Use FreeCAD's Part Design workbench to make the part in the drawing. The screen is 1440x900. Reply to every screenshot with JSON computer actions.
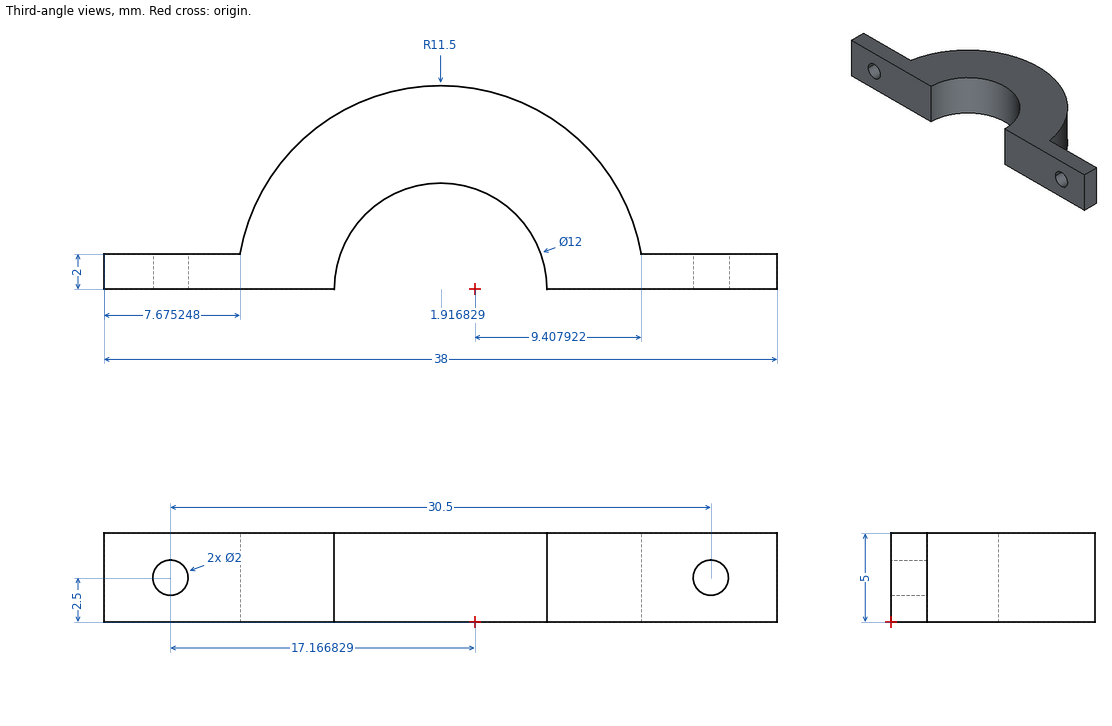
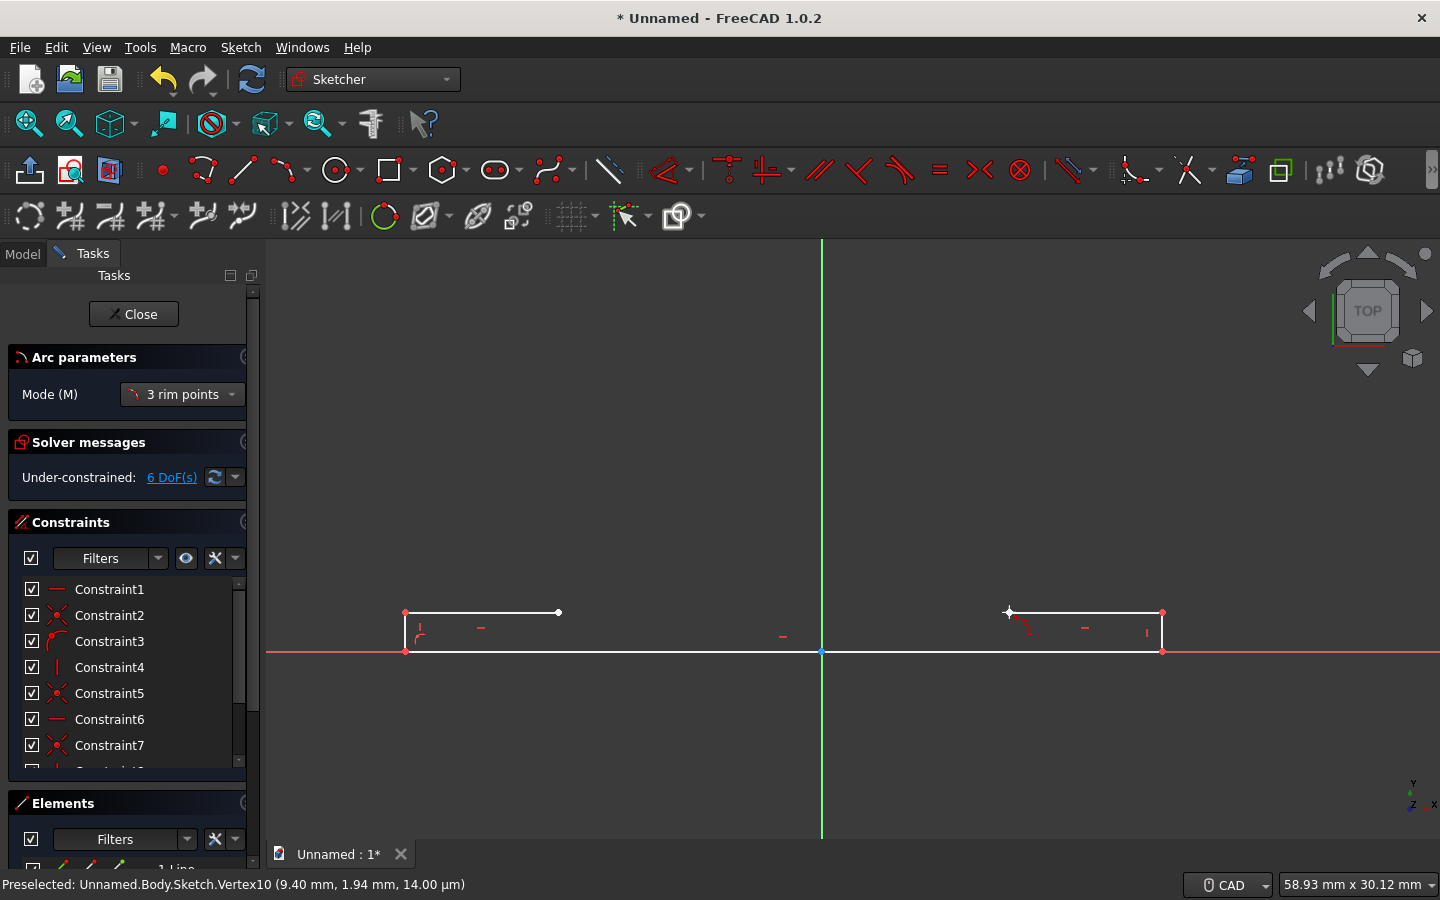
{"action": "left_click", "coordinate": [1009, 613]}
{"action": "left_click", "coordinate": [558, 613]}
{"action": "left_click", "coordinate": [783, 423]}
{"action": "key", "text": "Escape"}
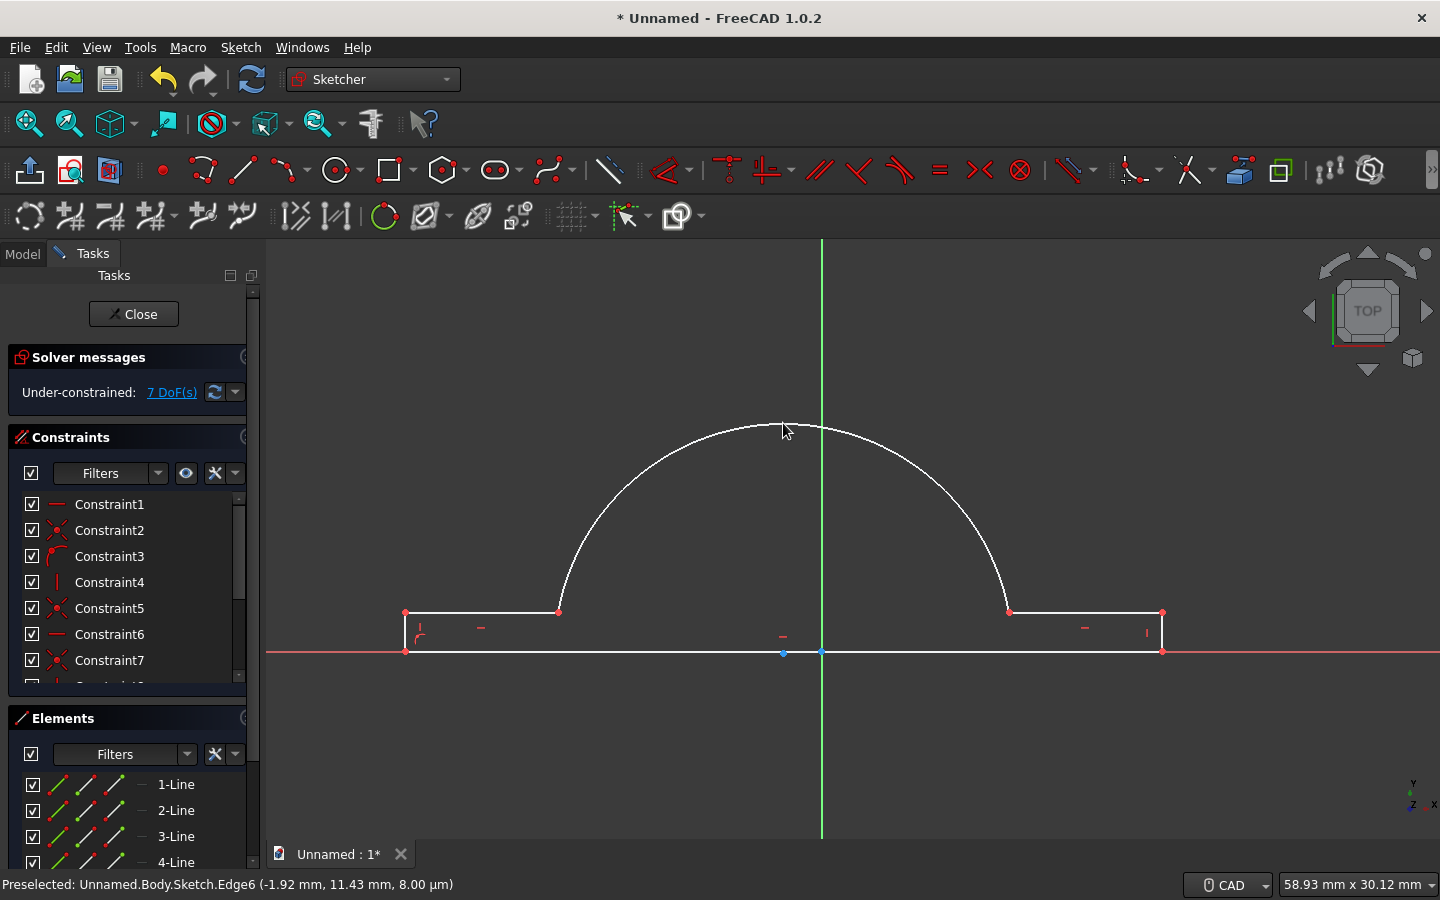
{"action": "left_click", "coordinate": [784, 653]}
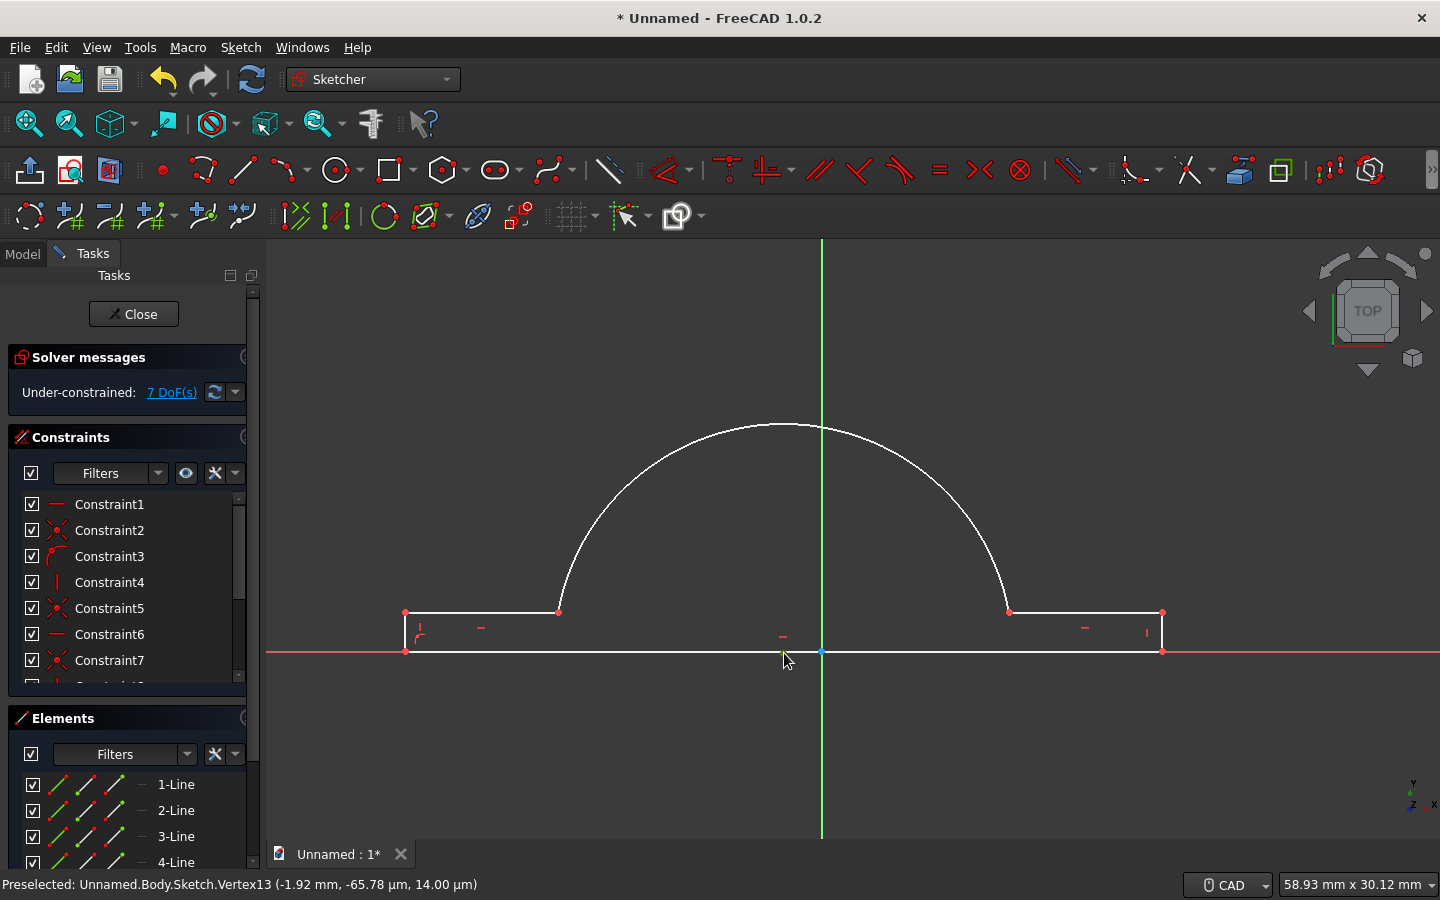
{"action": "left_click", "coordinate": [364, 652]}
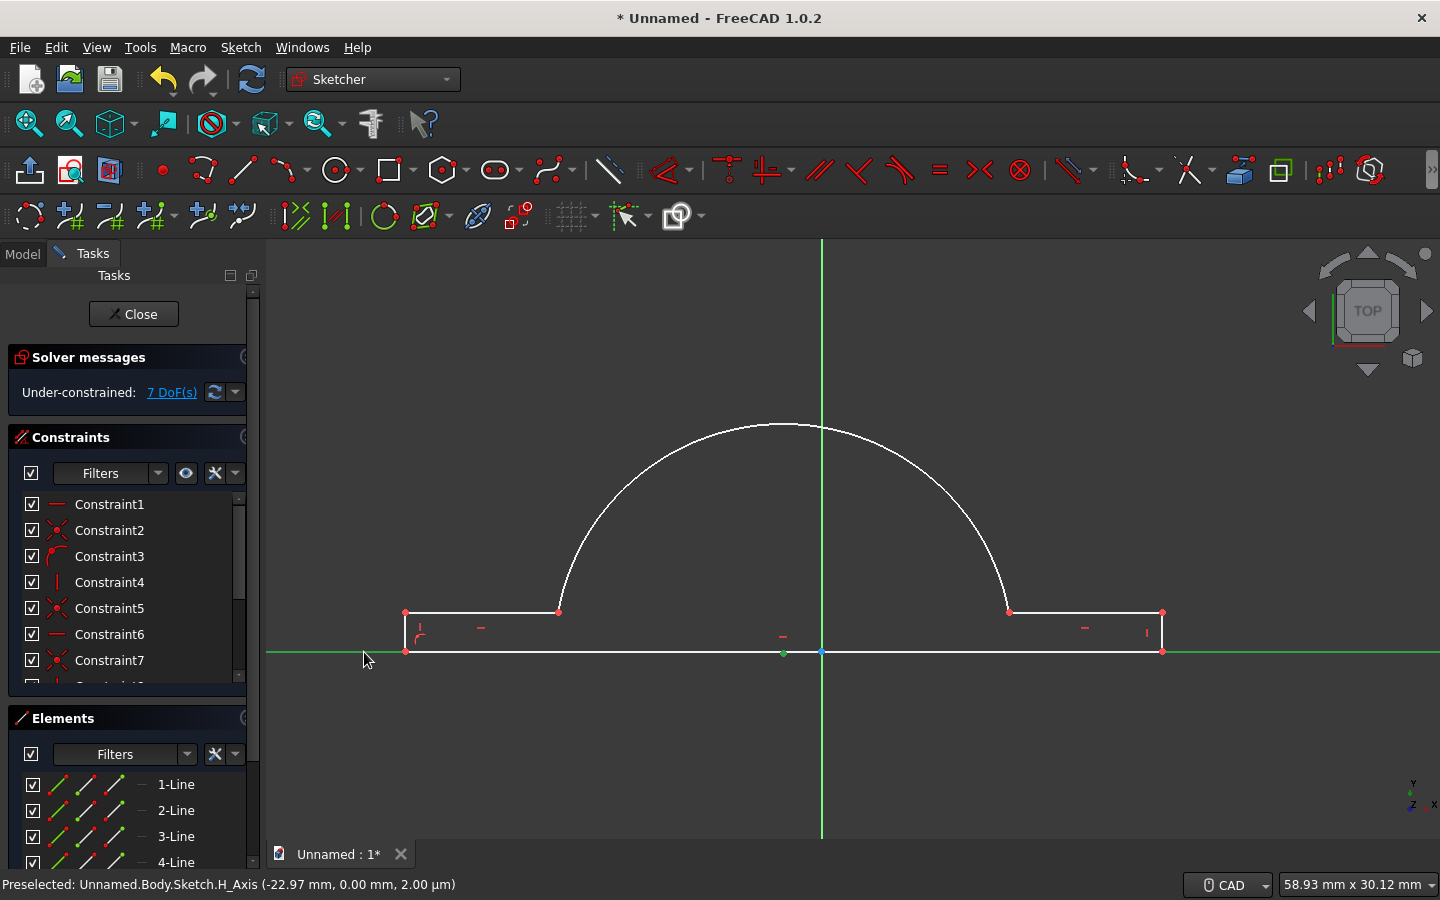
{"action": "left_click", "coordinate": [728, 170]}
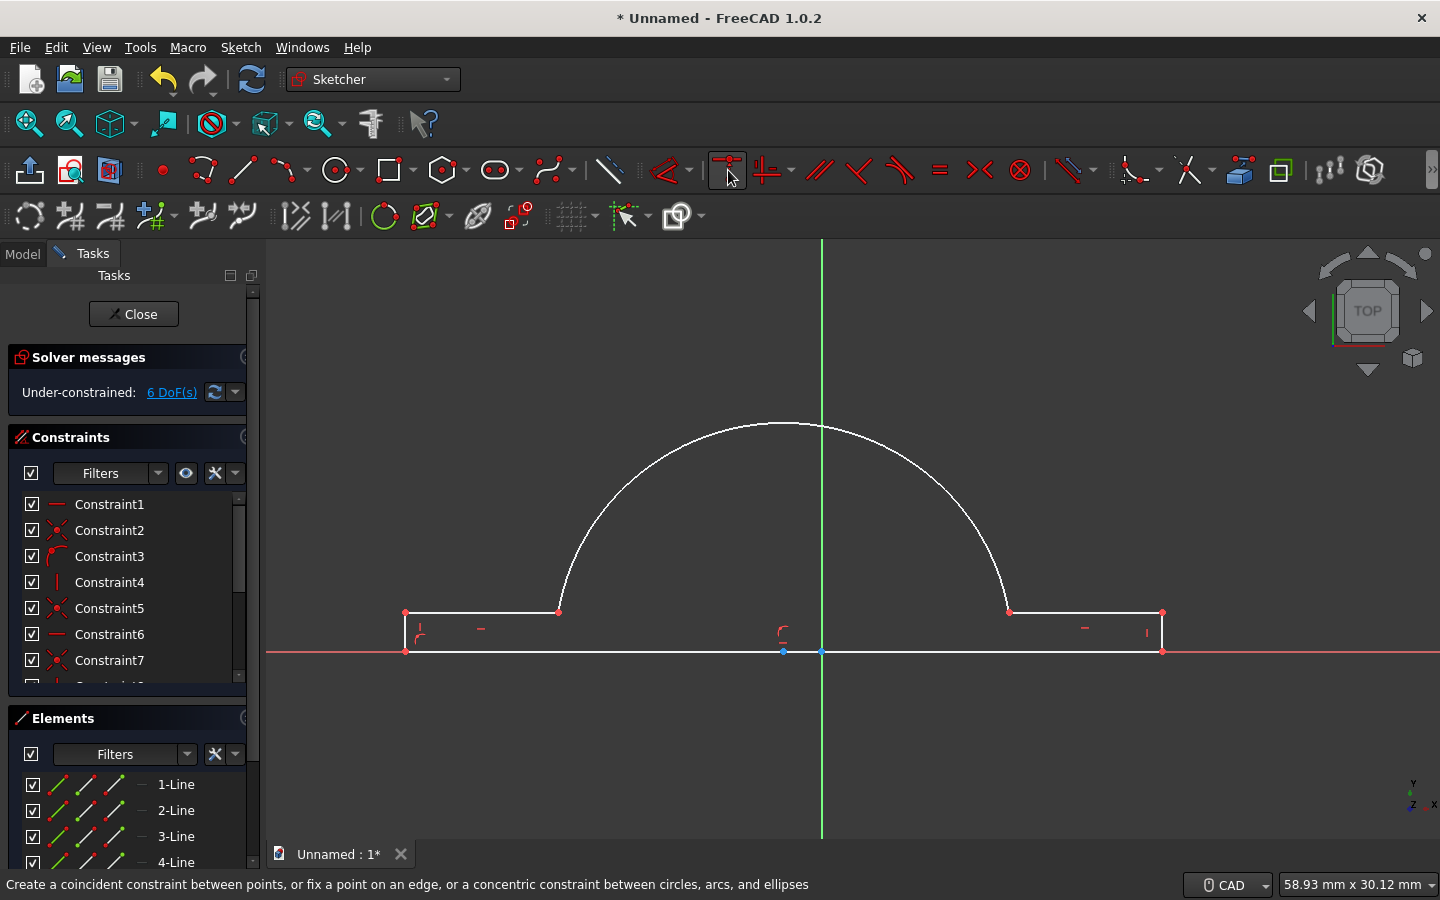
{"action": "key", "text": "d"}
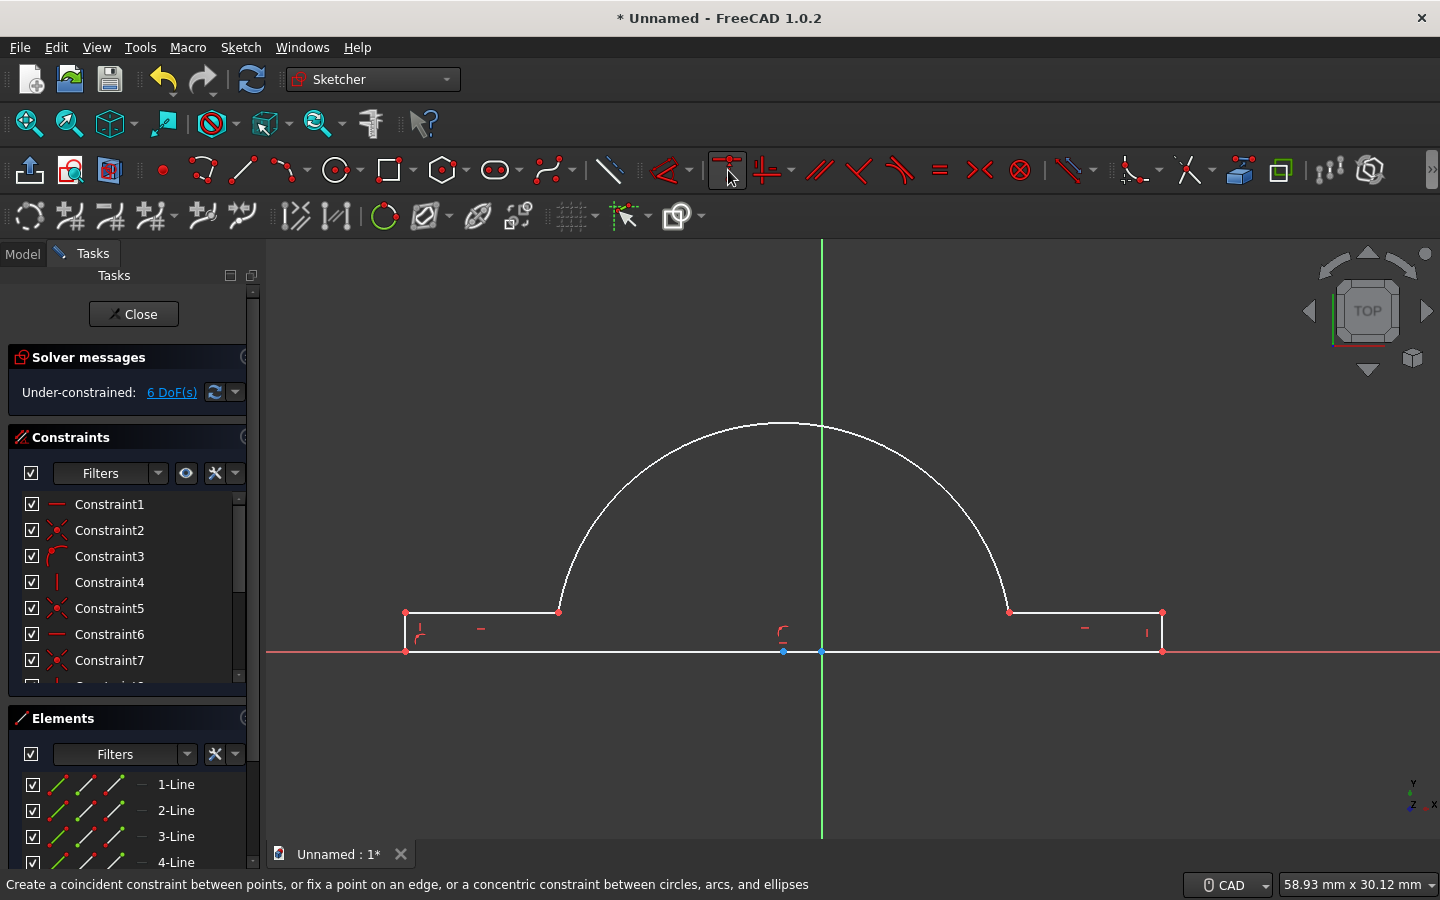
{"action": "left_click", "coordinate": [905, 458]}
{"action": "left_click", "coordinate": [922, 431]}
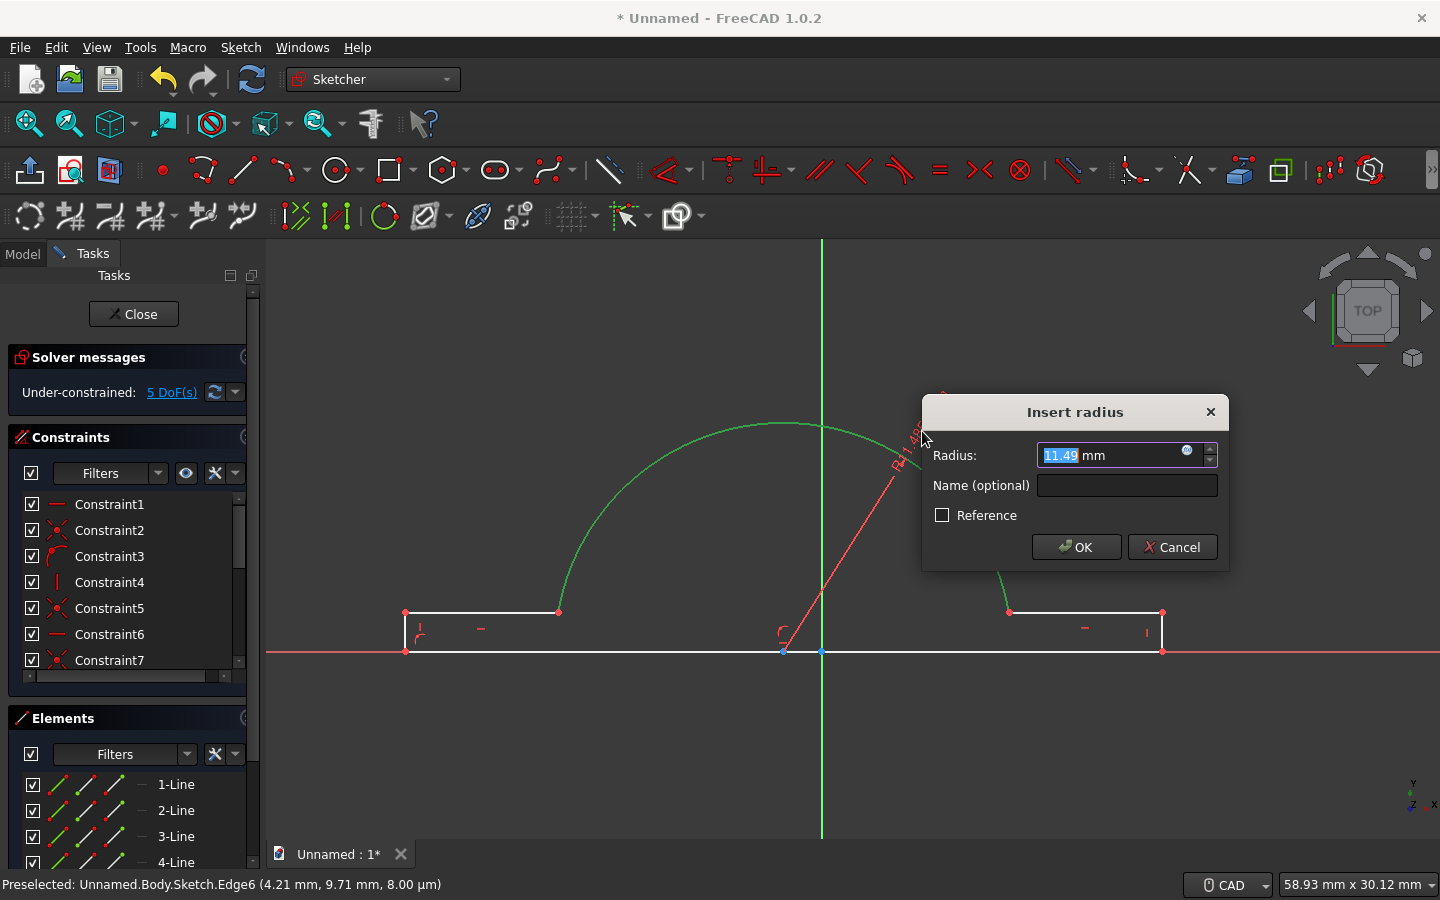
{"action": "type", "text": "11.5"}
{"action": "key", "text": "Return"}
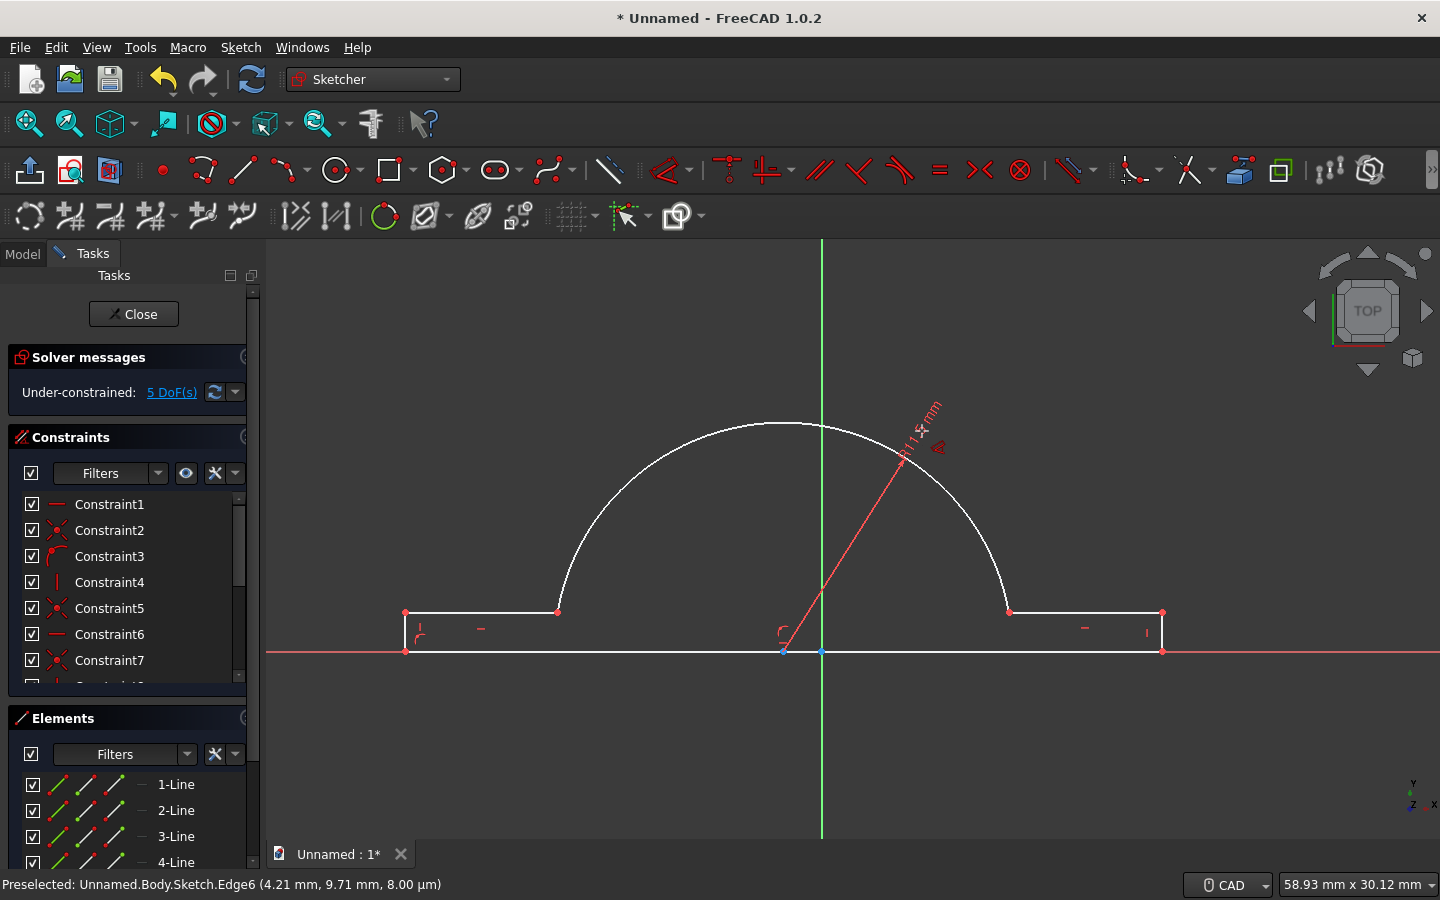
{"action": "left_click", "coordinate": [405, 625]}
{"action": "left_click", "coordinate": [371, 632]}